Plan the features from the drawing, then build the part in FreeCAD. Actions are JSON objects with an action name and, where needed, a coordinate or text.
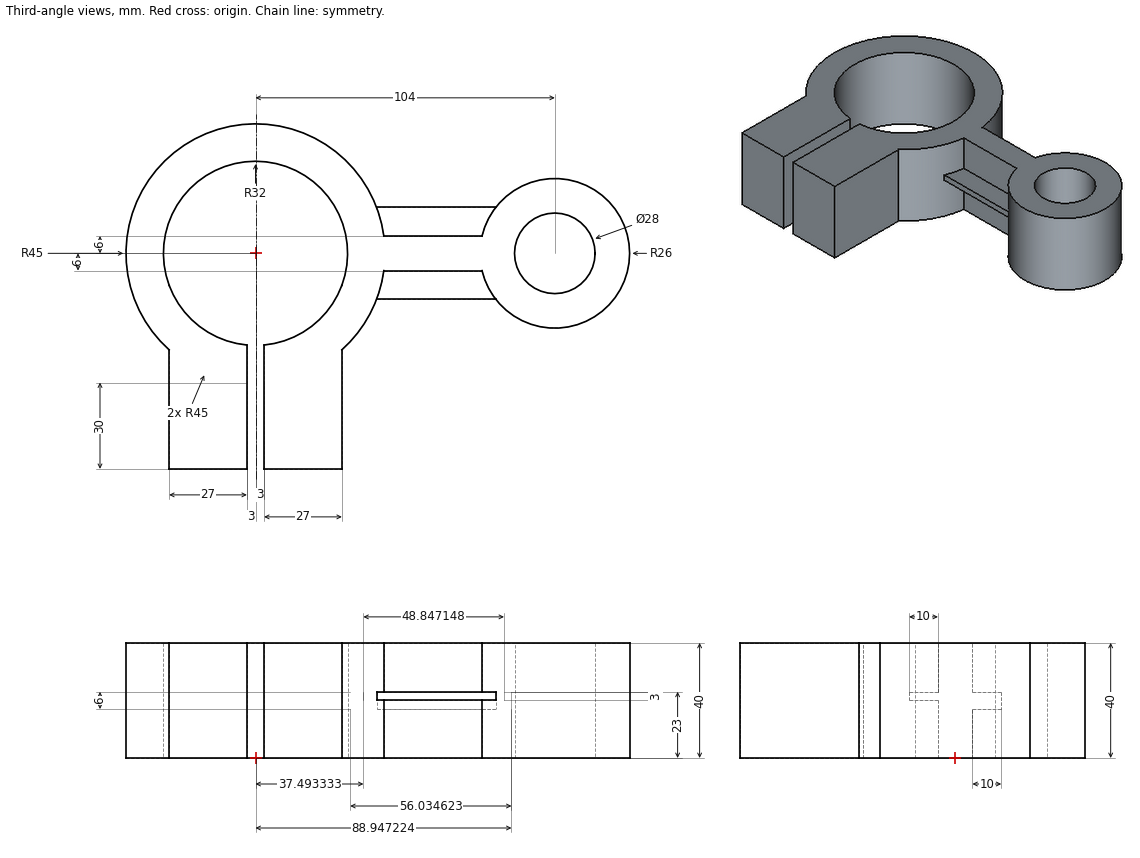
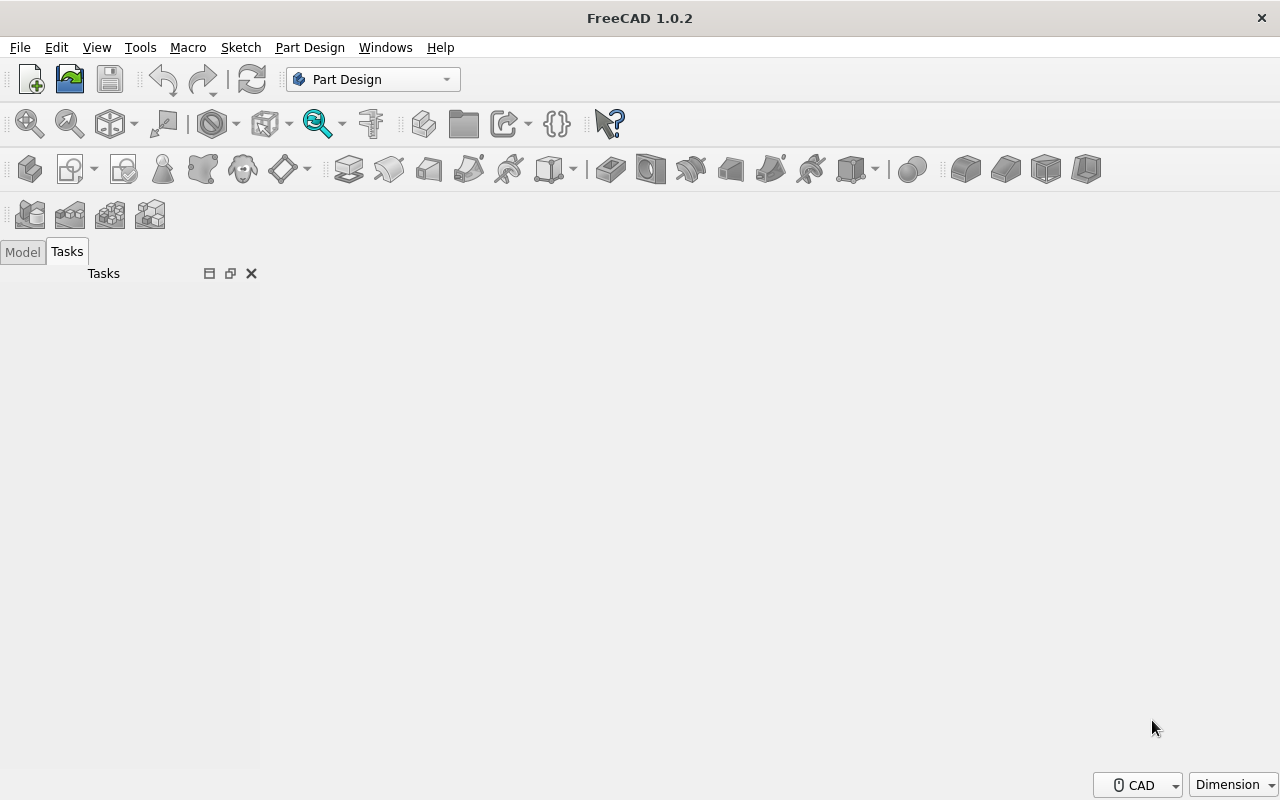
{"action": "key", "text": "ctrl+n"}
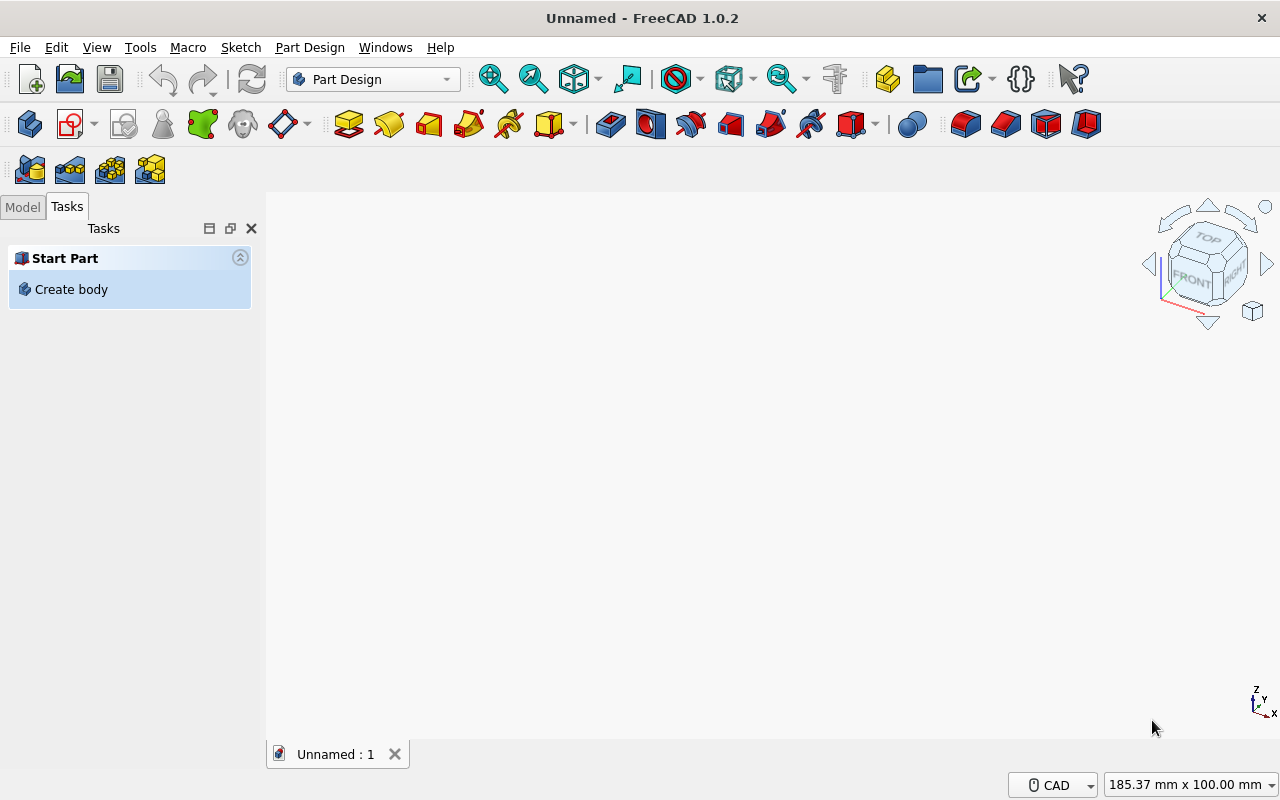
{"action": "left_click", "coordinate": [70, 124]}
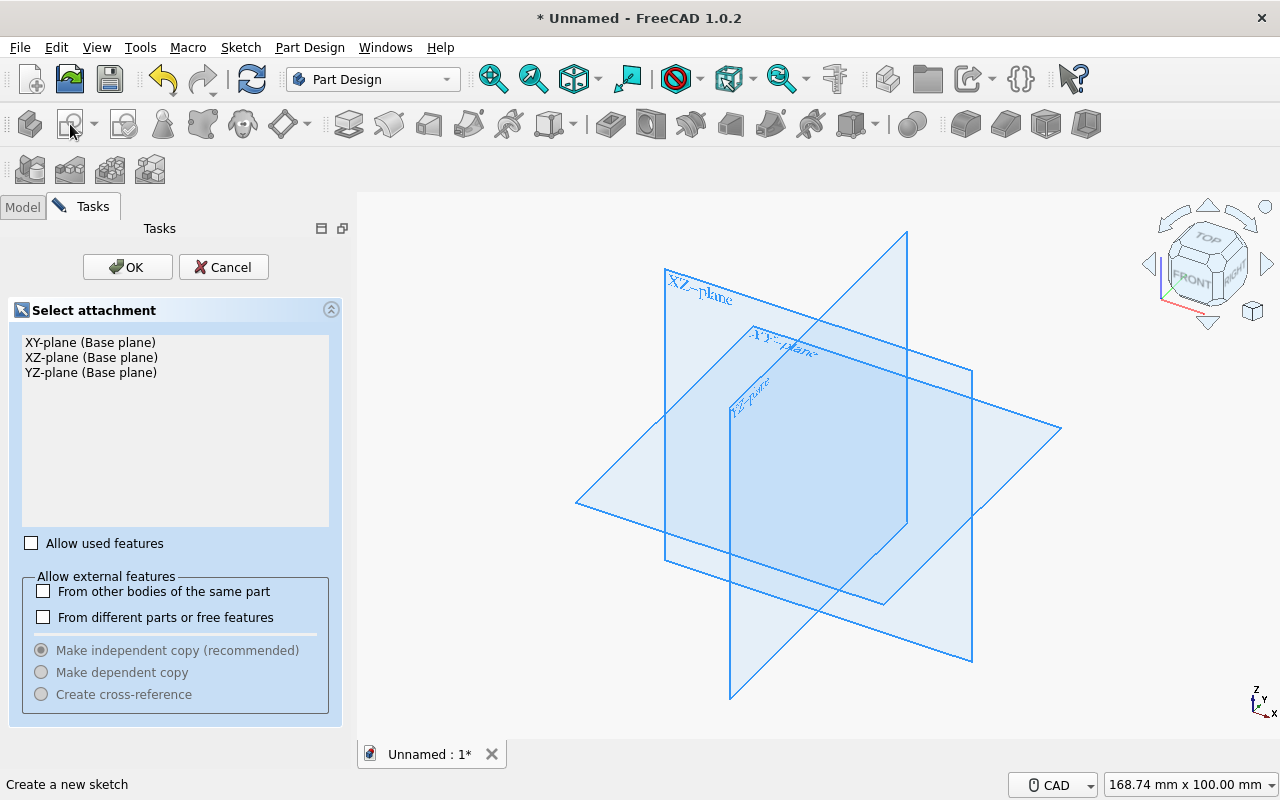
{"action": "left_click", "coordinate": [82, 342]}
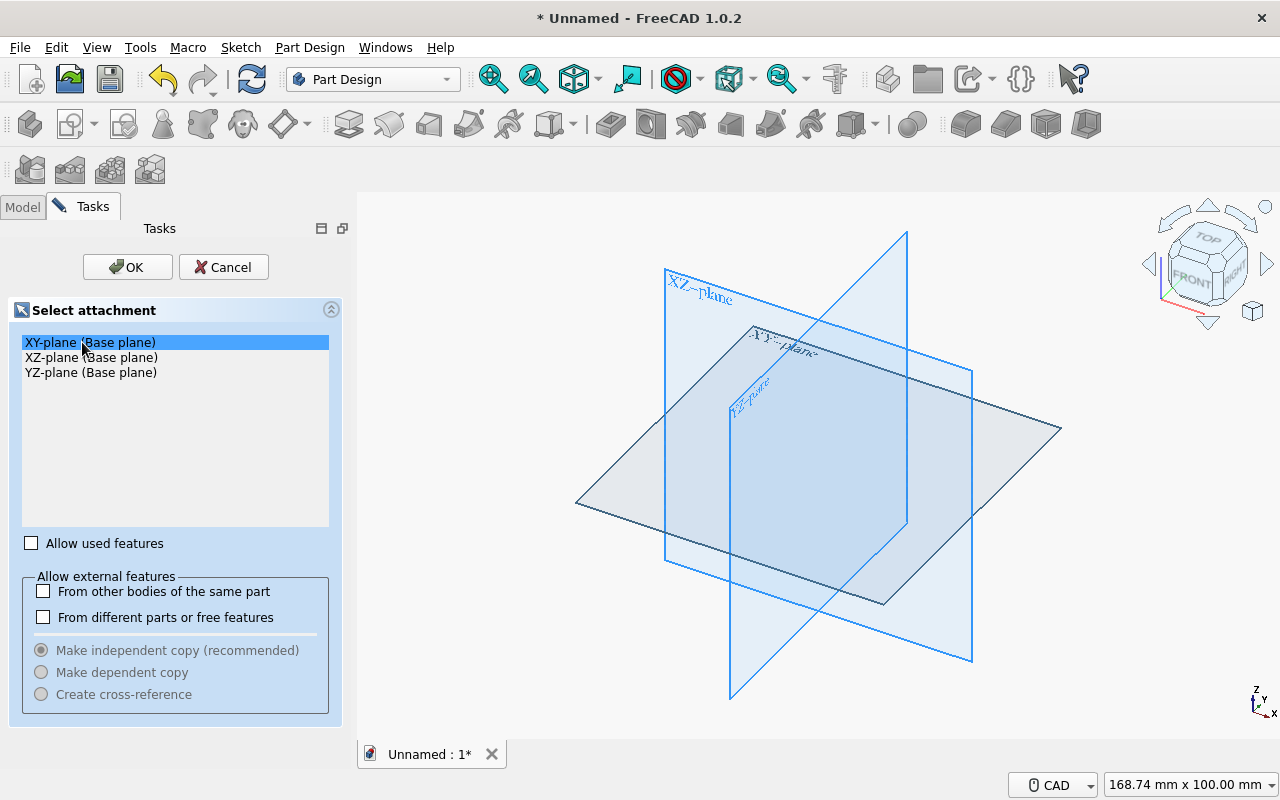
{"action": "left_click", "coordinate": [128, 267]}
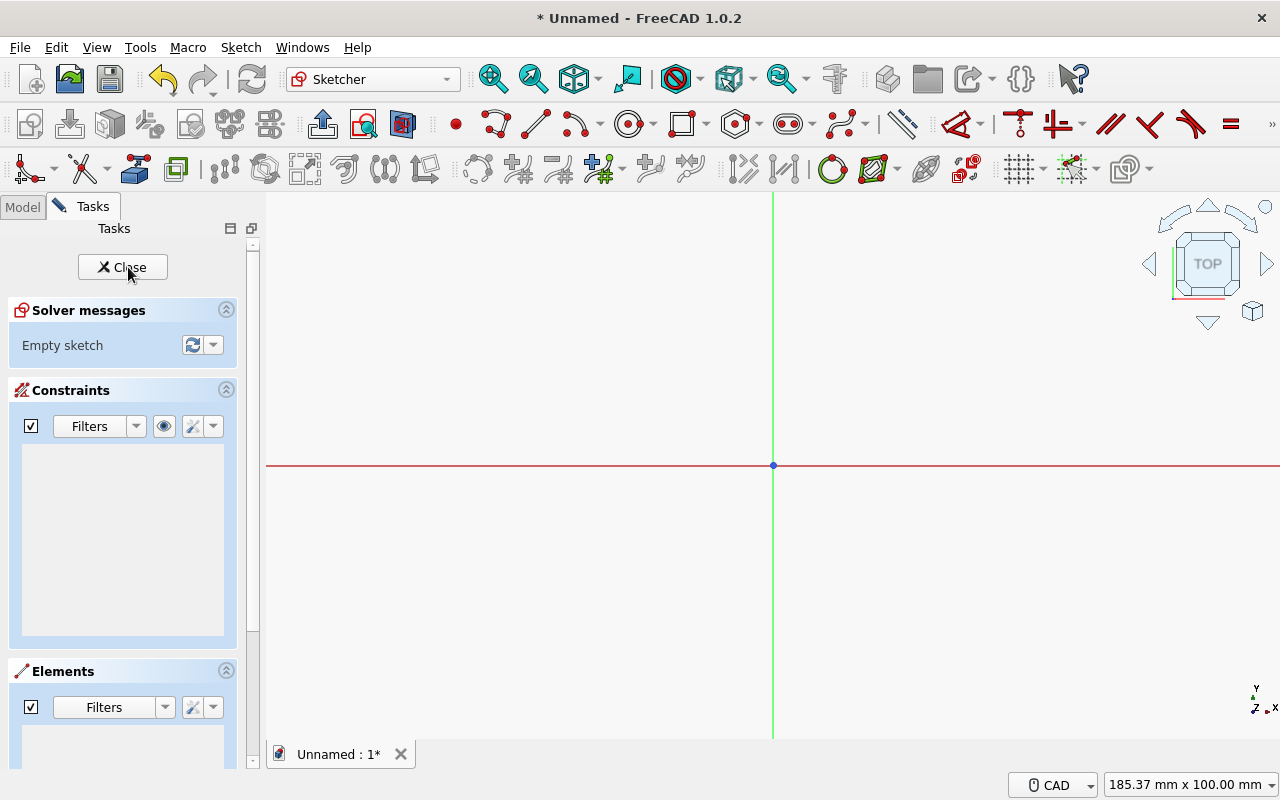
{"action": "scroll", "coordinate": [338, 466], "scroll_direction": "down", "scroll_amount": 3}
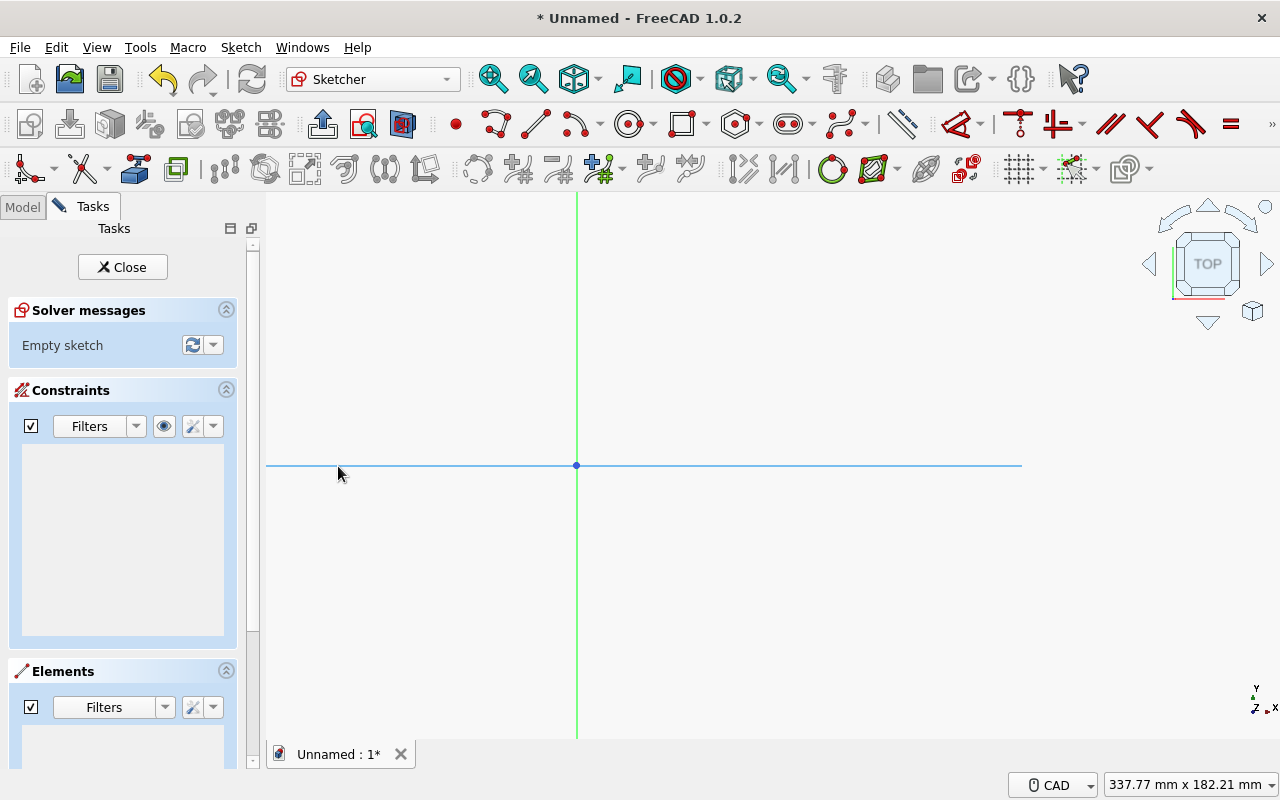
{"action": "key", "text": "g l"}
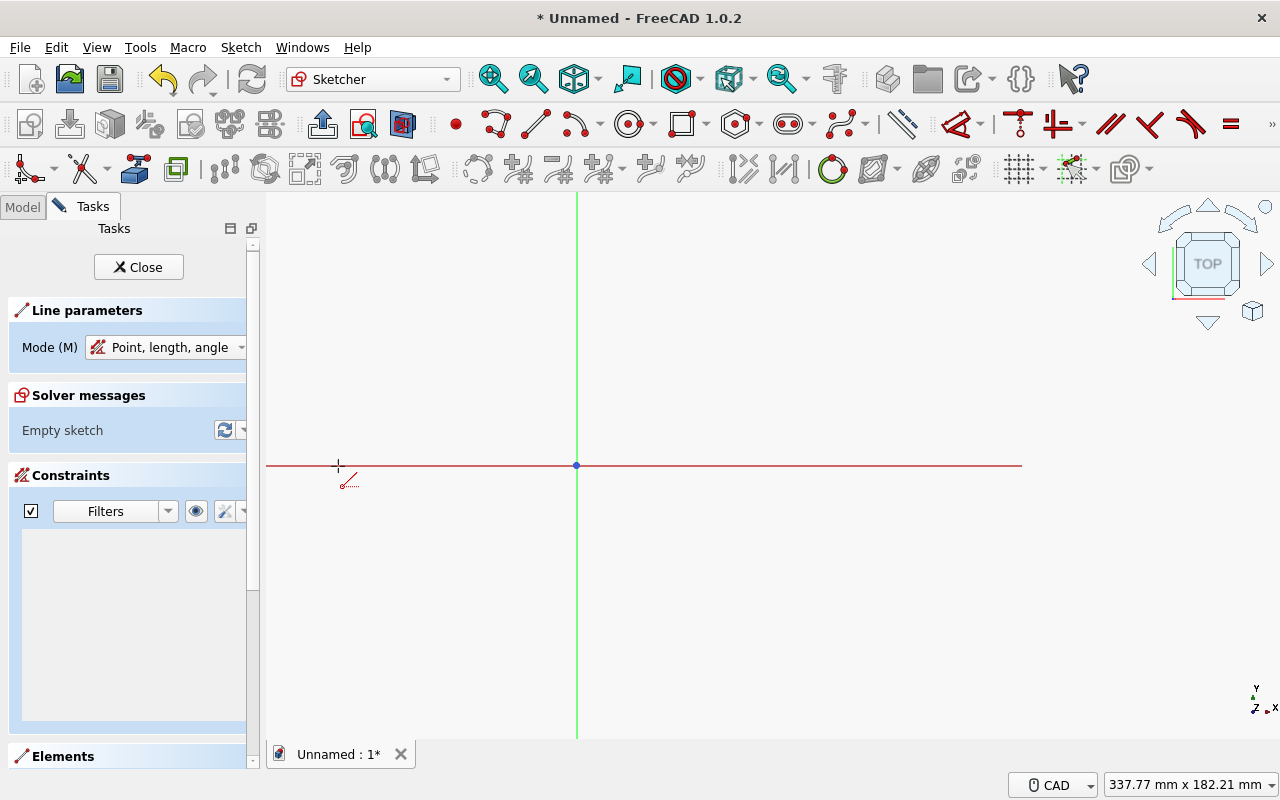
{"action": "left_click", "coordinate": [813, 448]}
{"action": "left_click", "coordinate": [711, 448]}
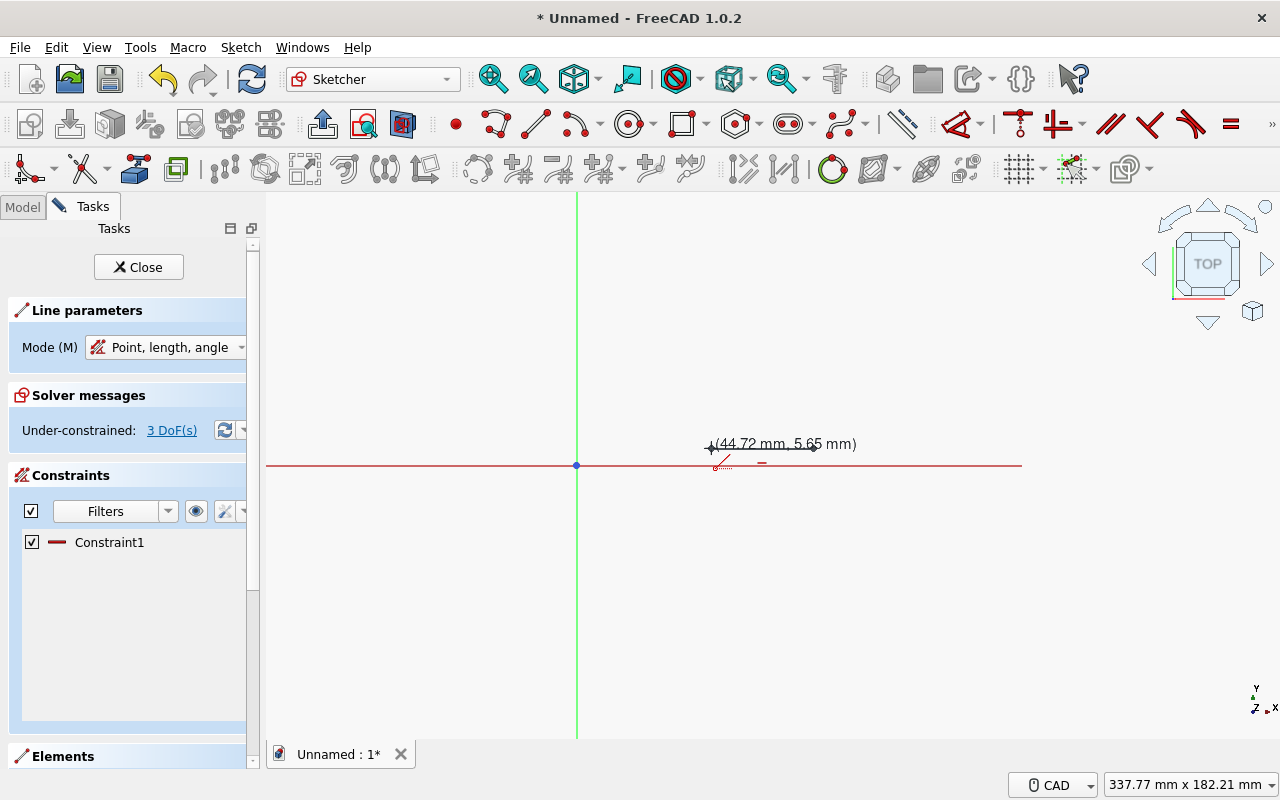
{"action": "left_click", "coordinate": [711, 484]}
{"action": "left_click", "coordinate": [813, 484]}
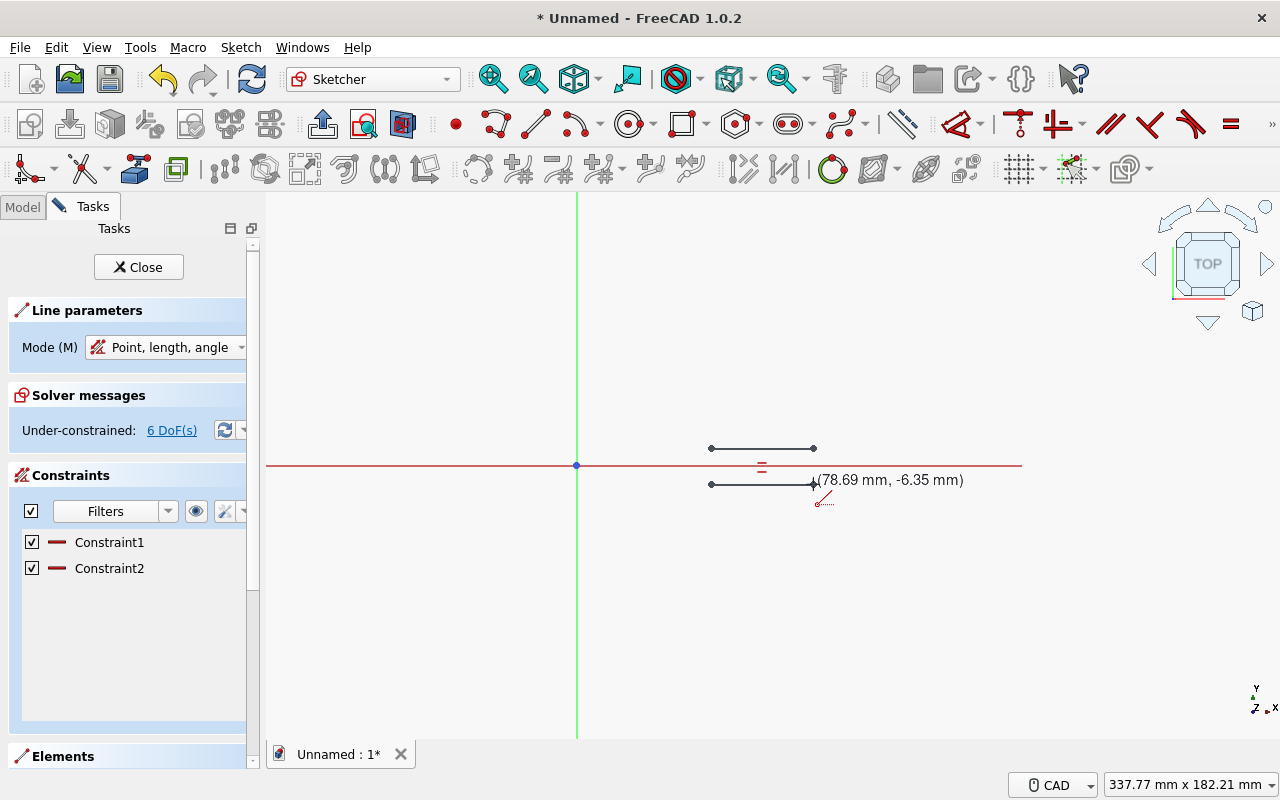
{"action": "key", "text": "g 3 a"}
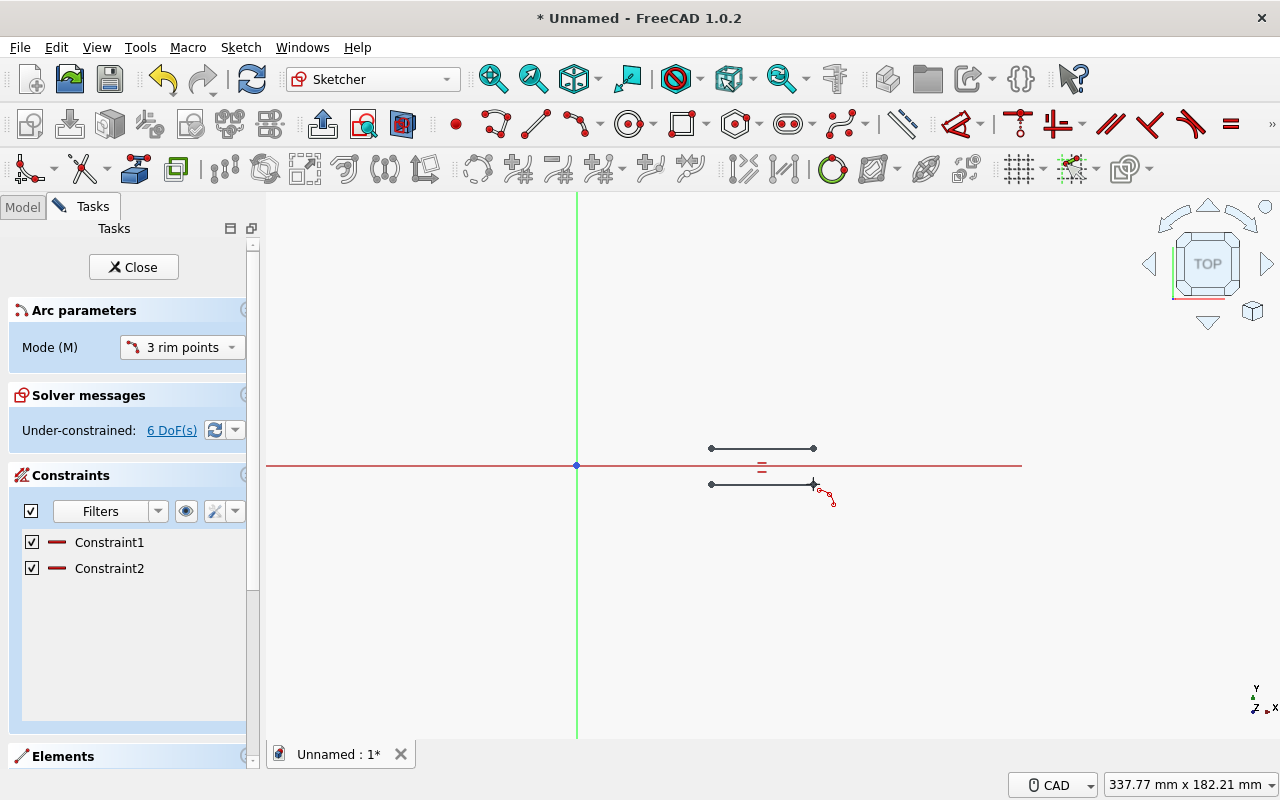
{"action": "left_click", "coordinate": [711, 449]}
{"action": "left_click", "coordinate": [711, 485]}
{"action": "left_click", "coordinate": [465, 389]}